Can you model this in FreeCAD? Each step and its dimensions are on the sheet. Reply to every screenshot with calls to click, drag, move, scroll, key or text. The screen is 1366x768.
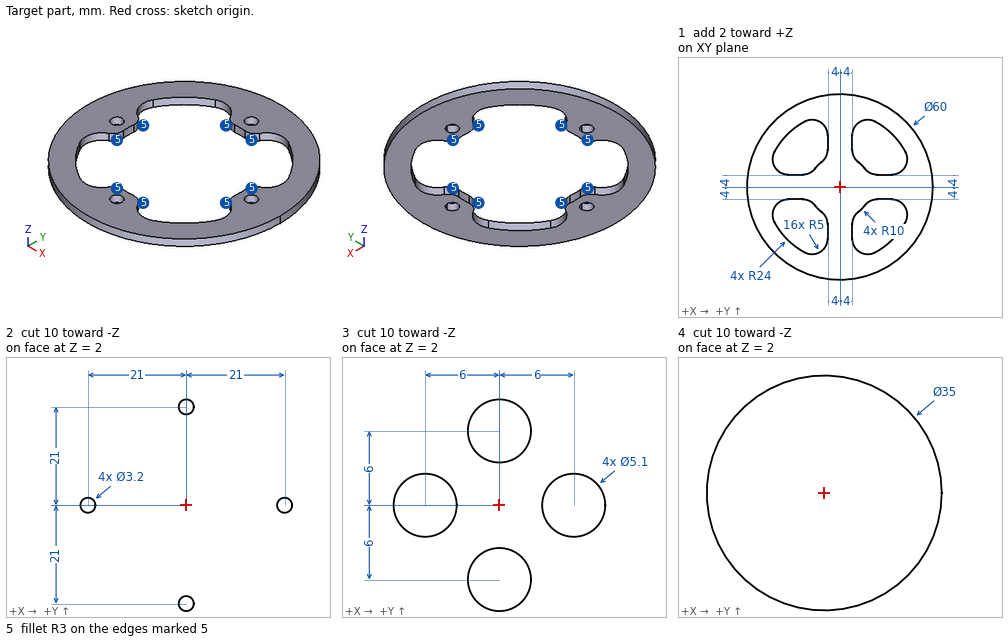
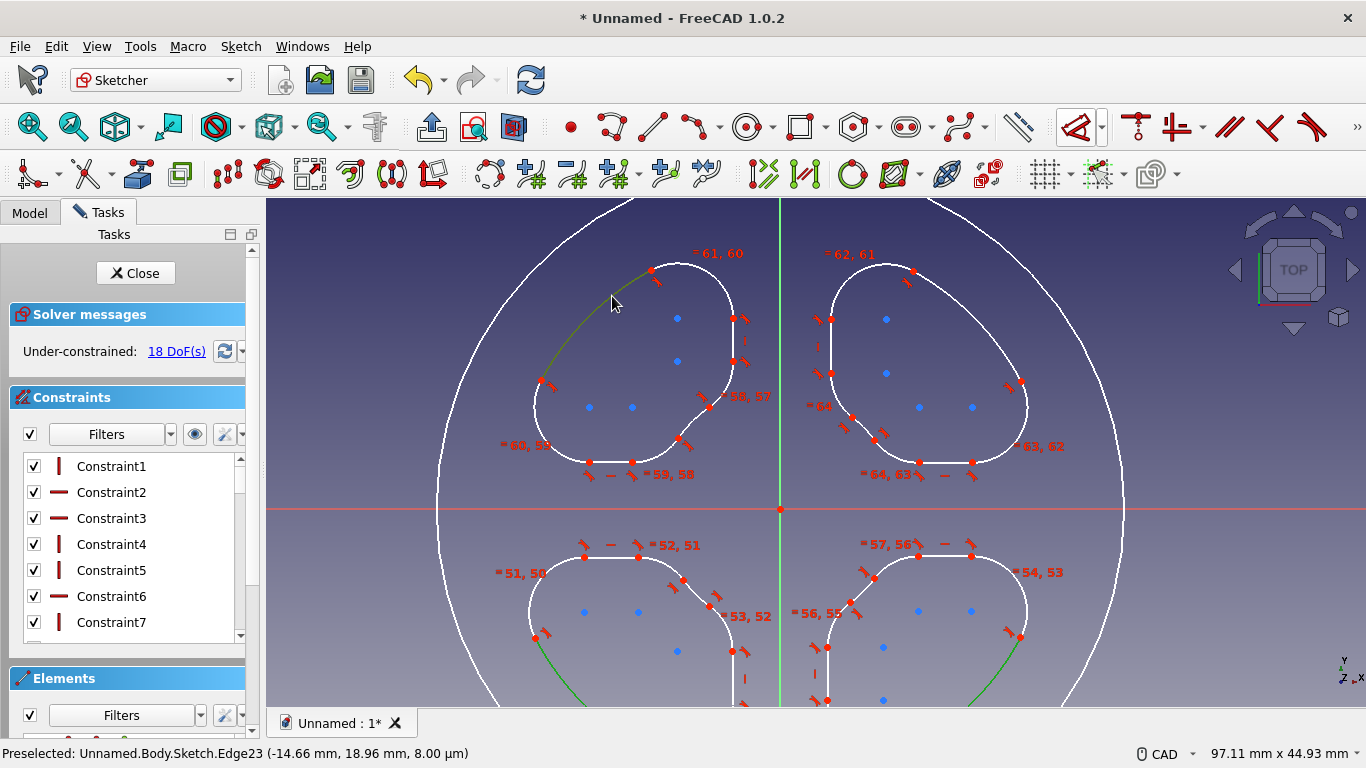
click(996, 342)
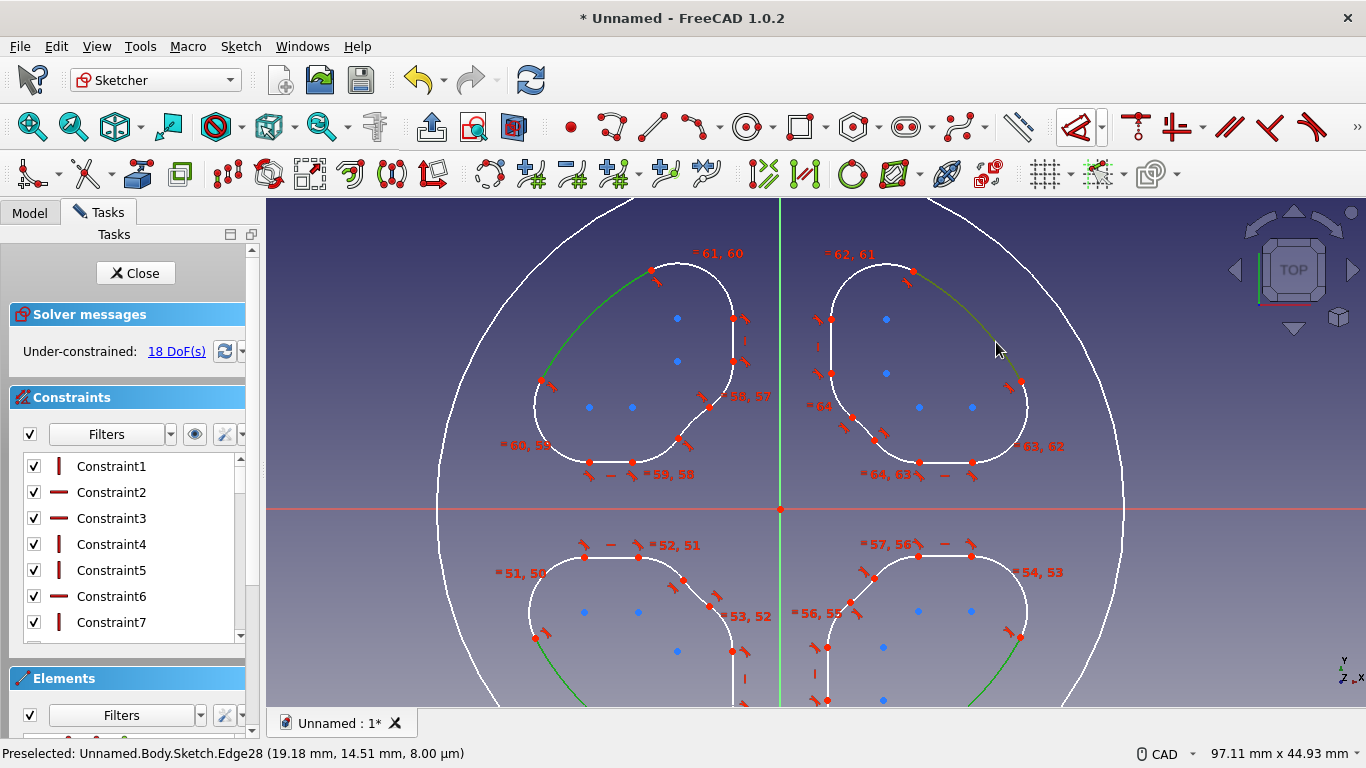
key(e)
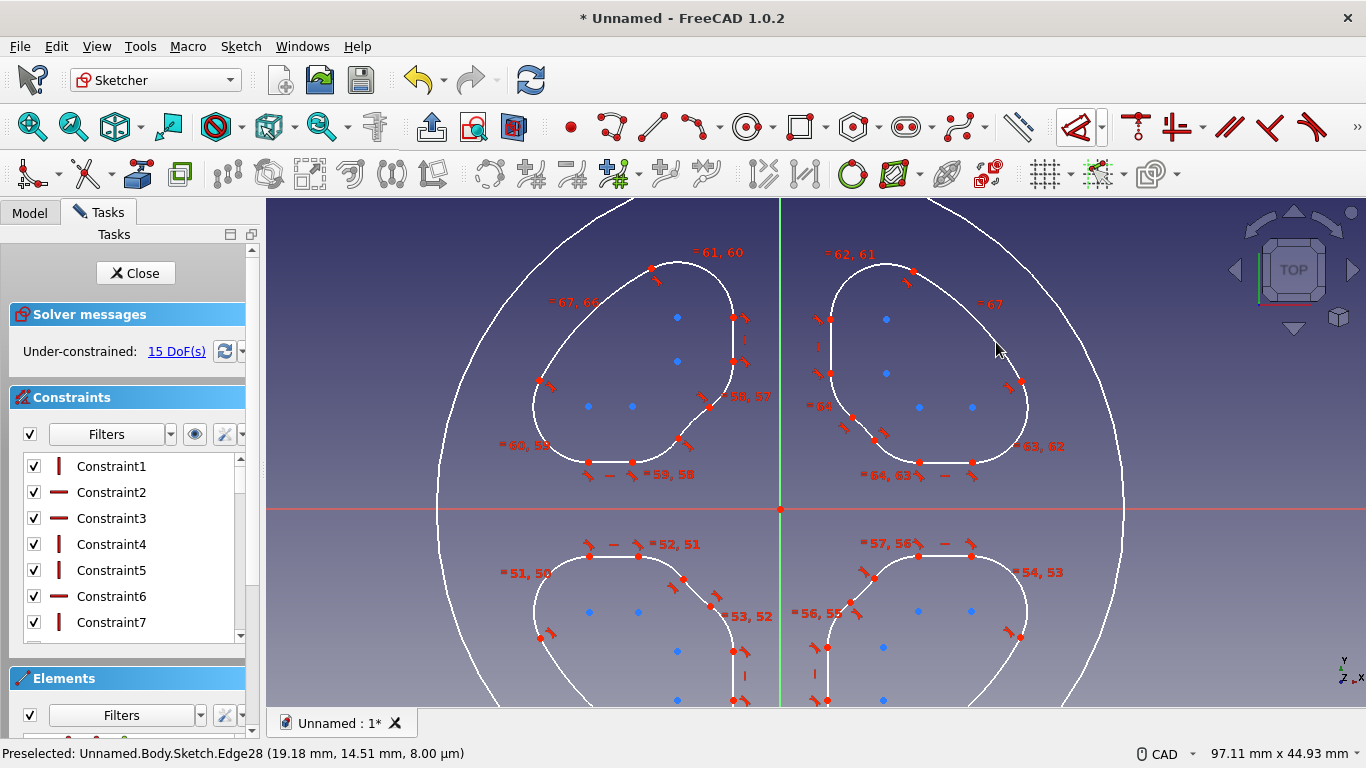
scroll(691, 588, up, 2)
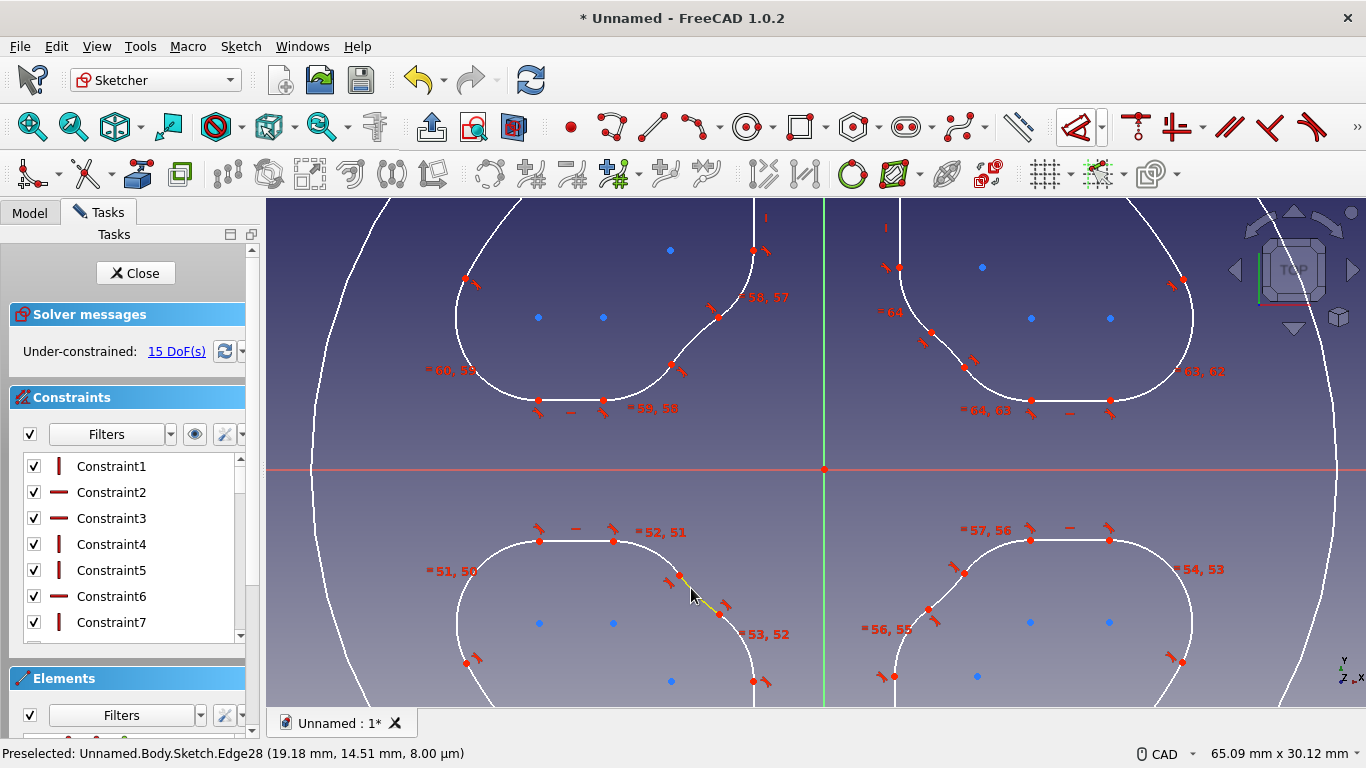
click(690, 588)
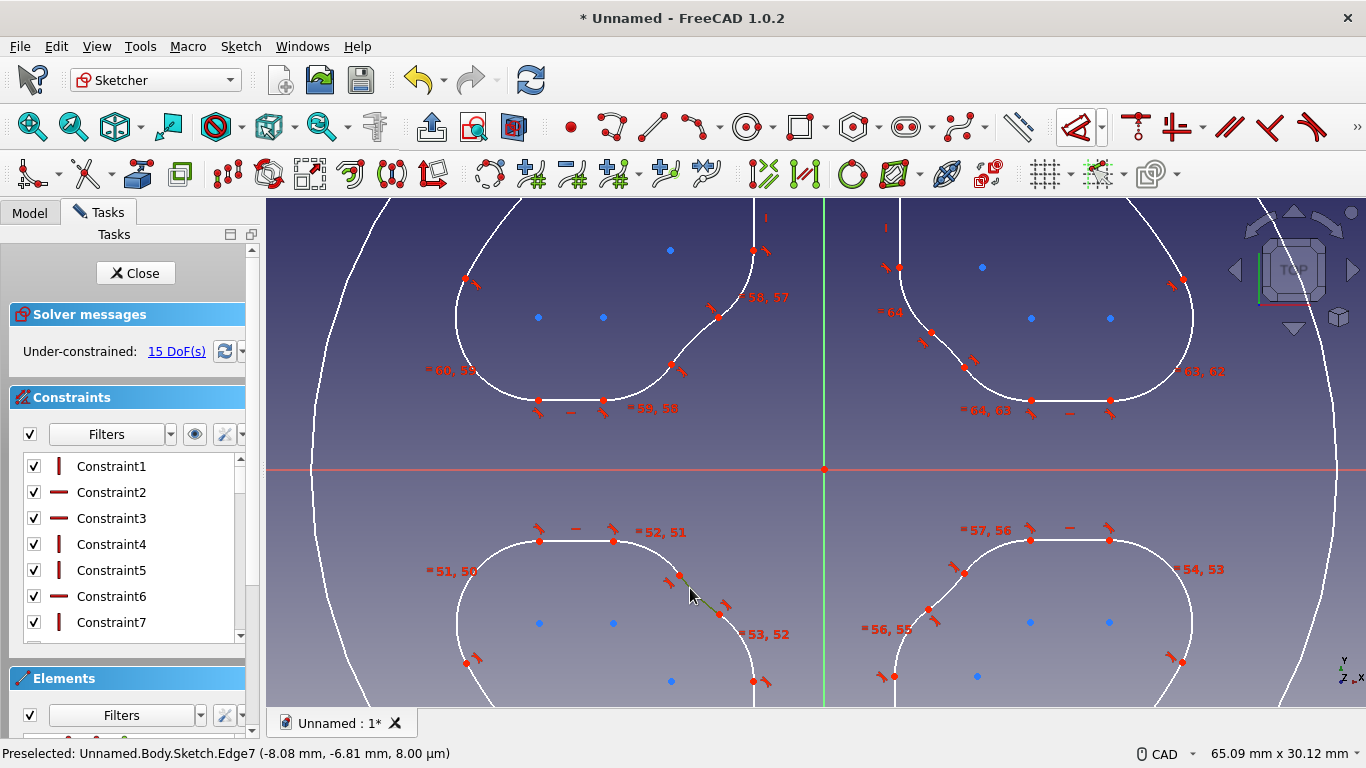
click(940, 600)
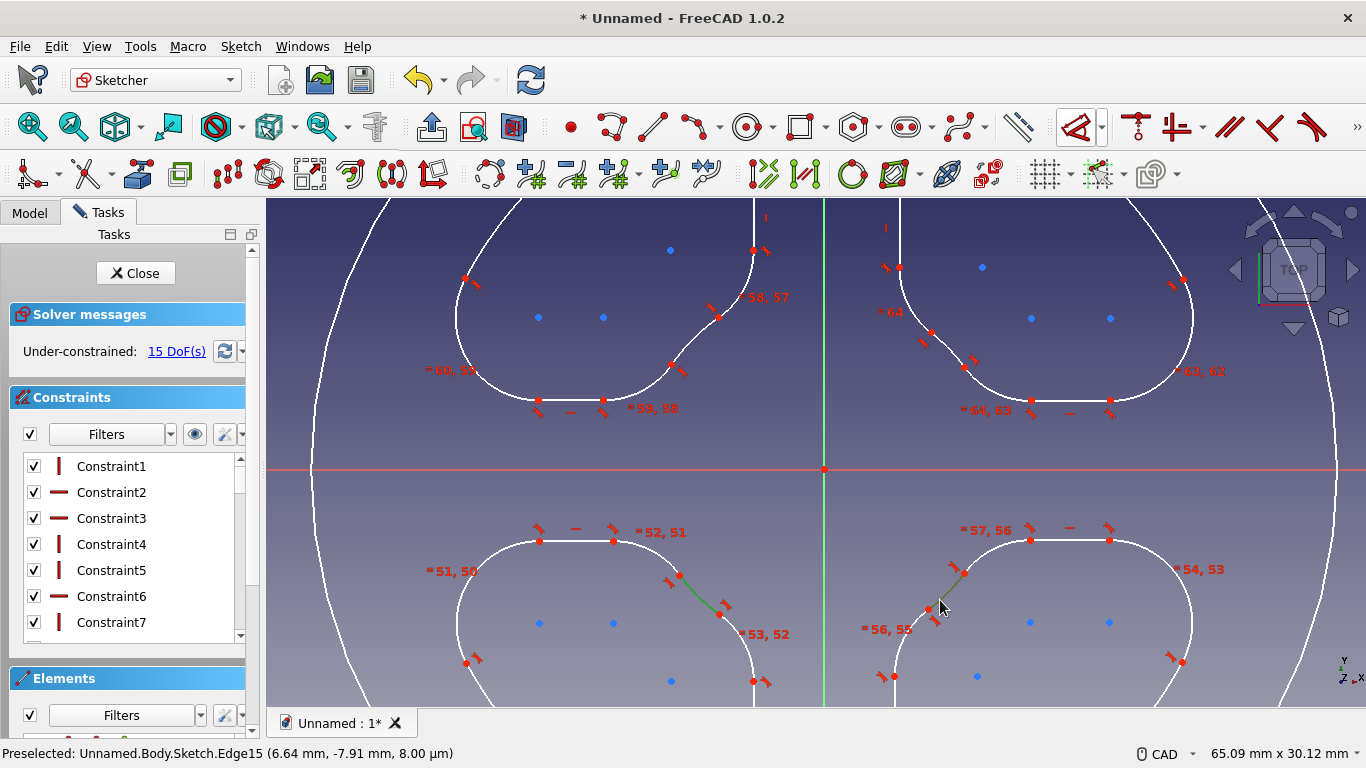
click(703, 330)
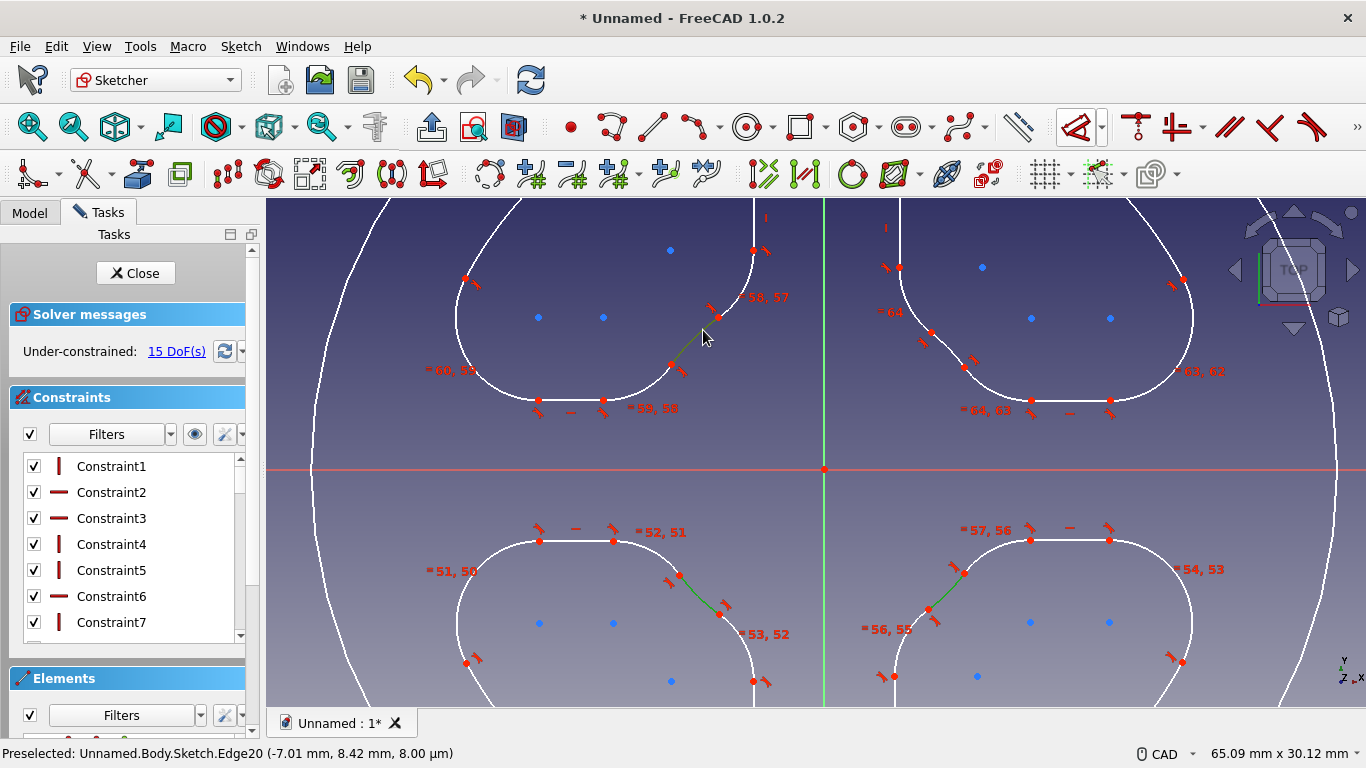
click(955, 356)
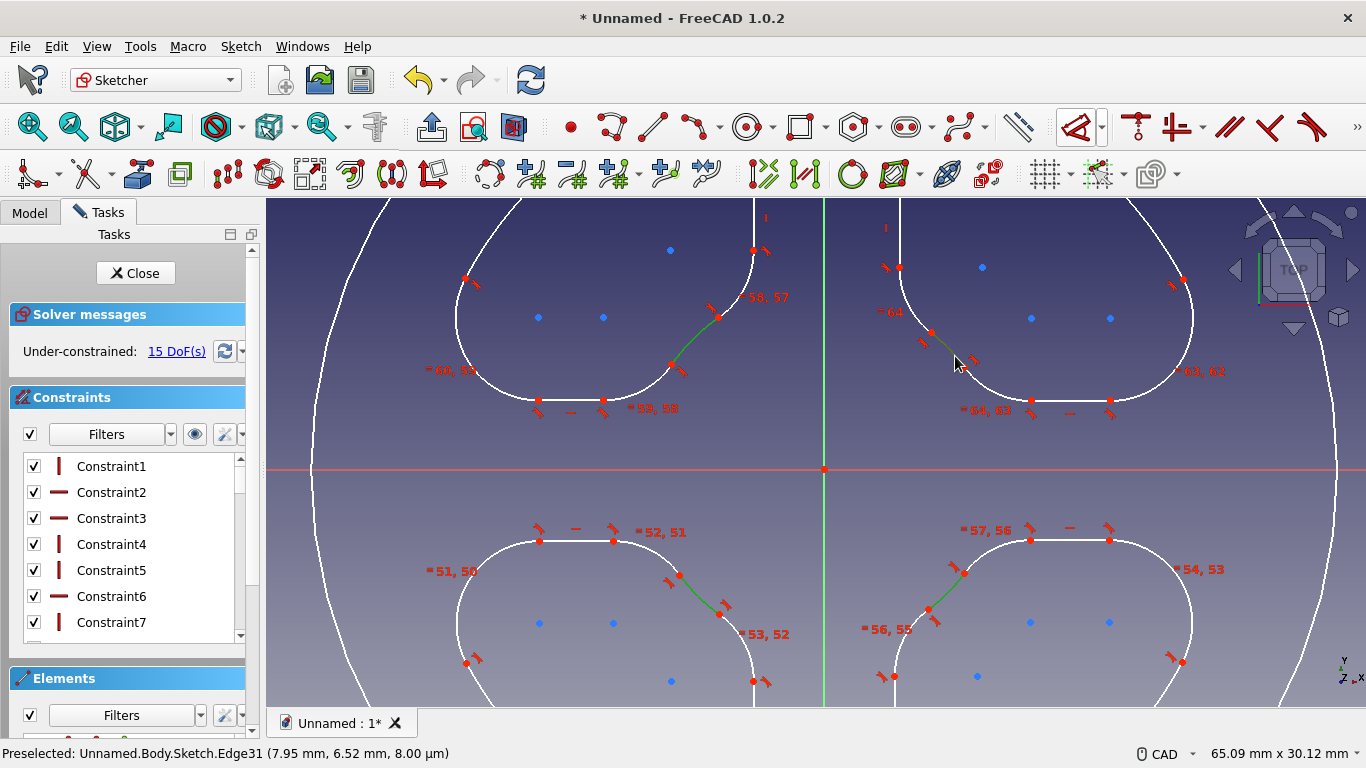
key(e)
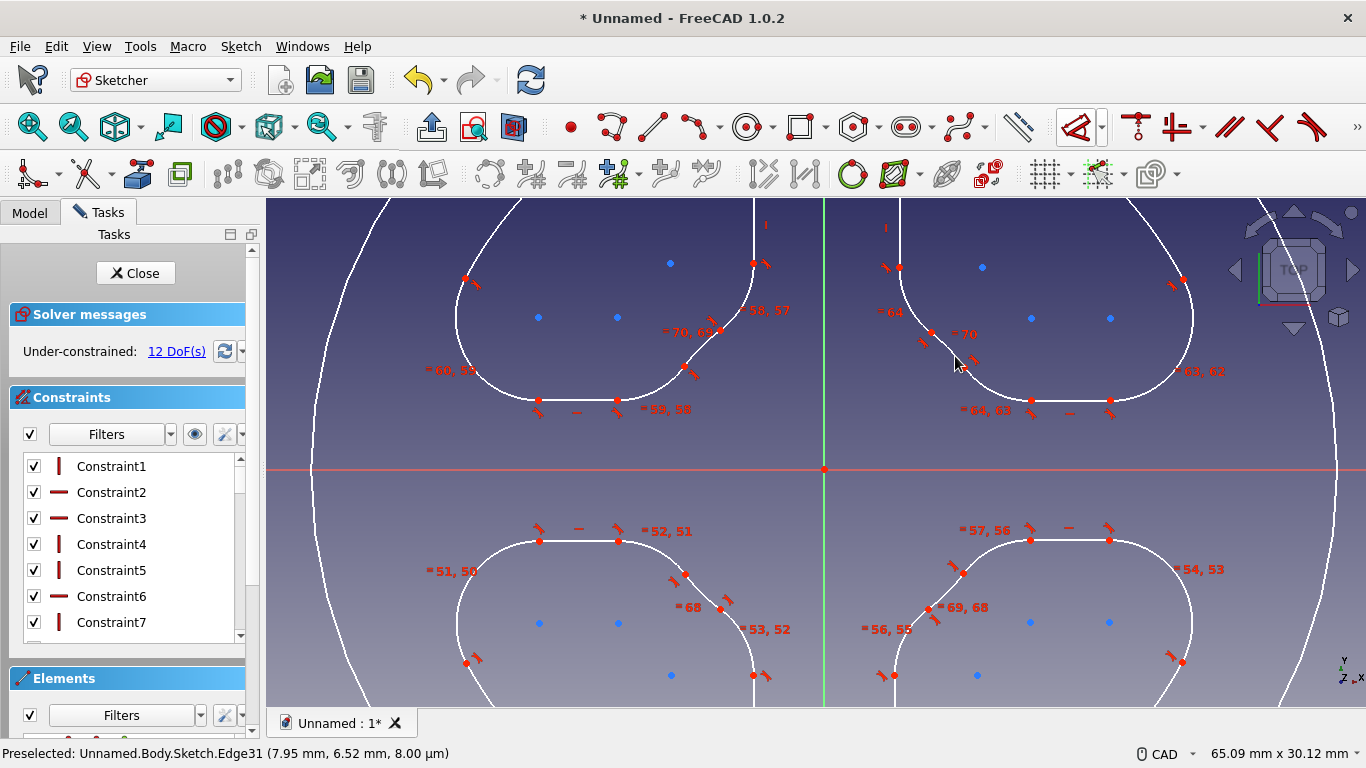
key(d)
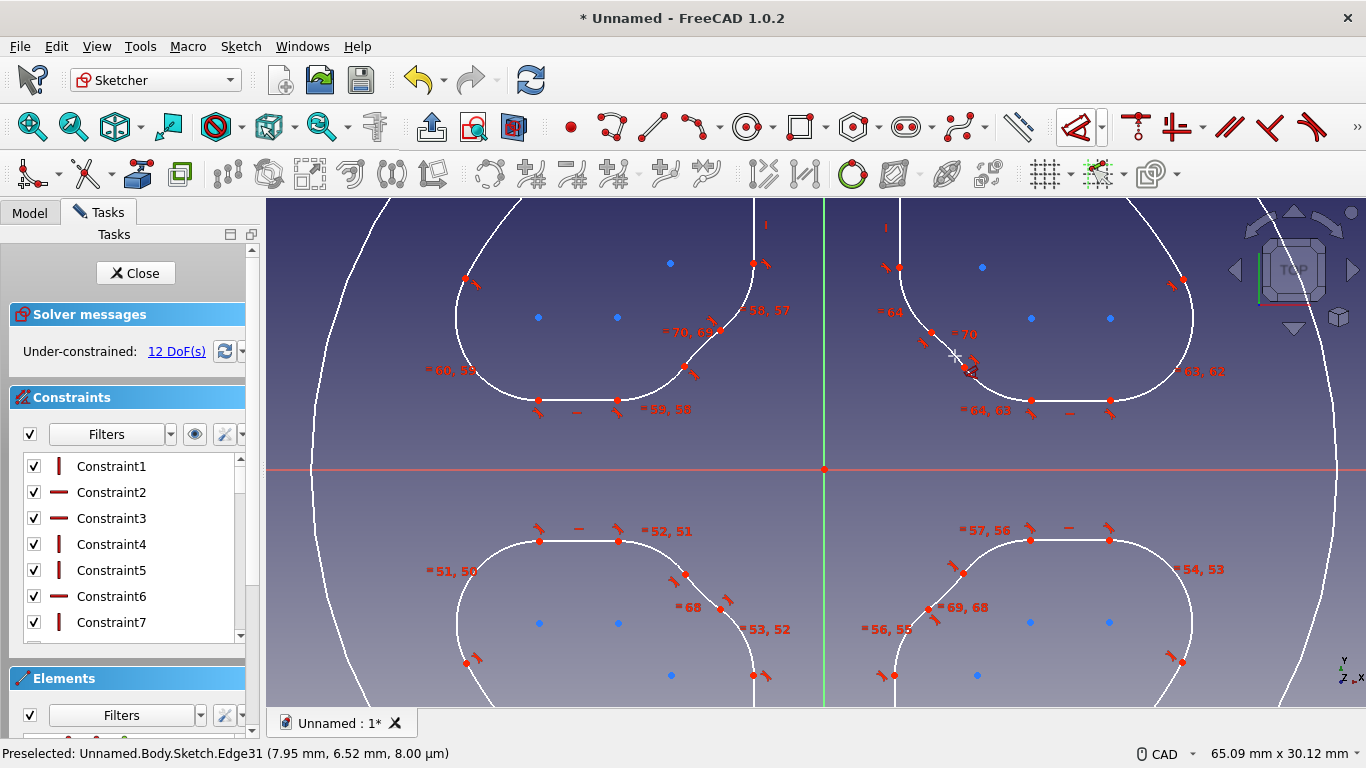
scroll(714, 445, down, 6)